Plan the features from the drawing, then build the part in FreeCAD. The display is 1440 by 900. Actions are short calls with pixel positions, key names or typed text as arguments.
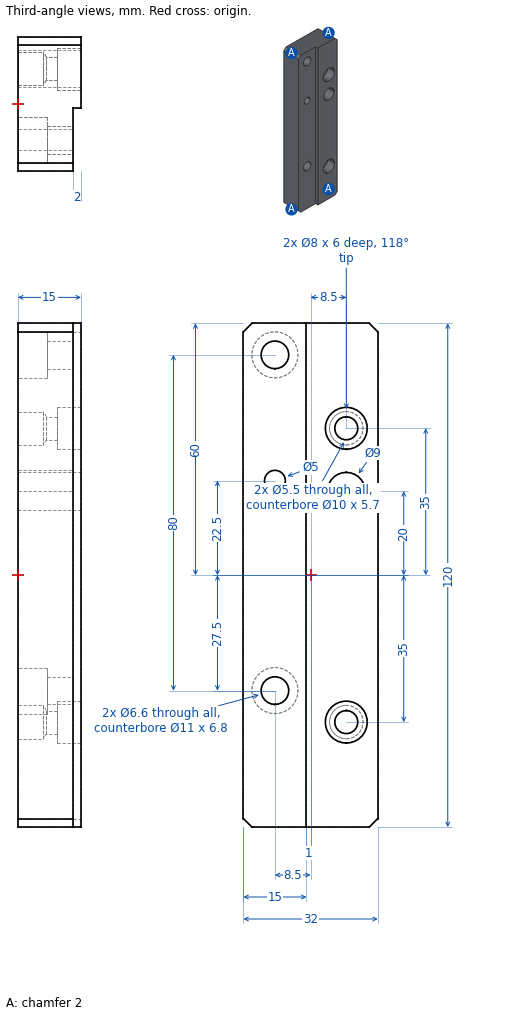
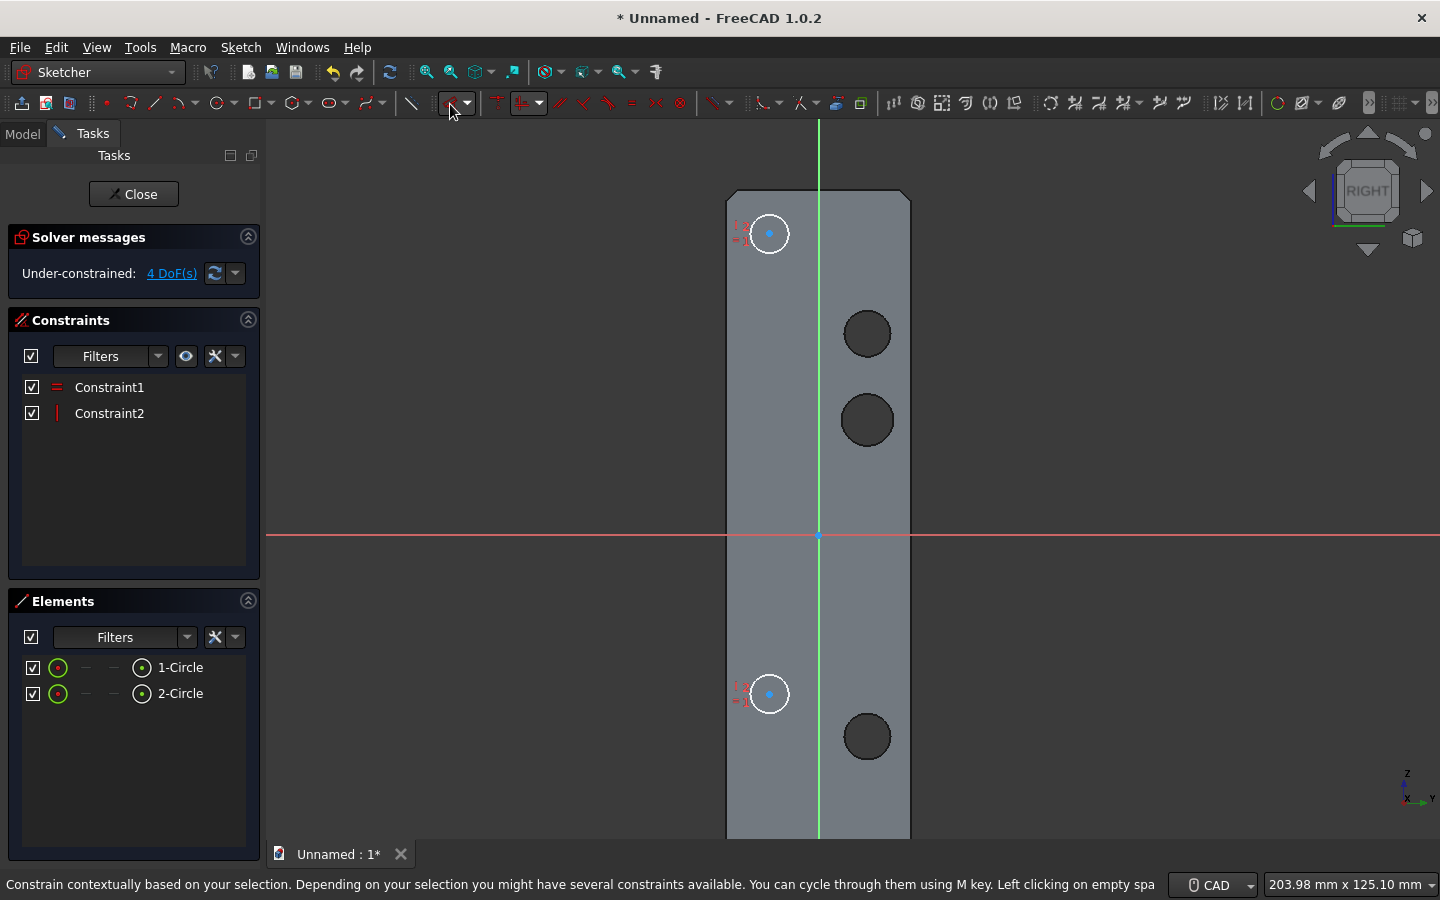
click(783, 681)
click(785, 646)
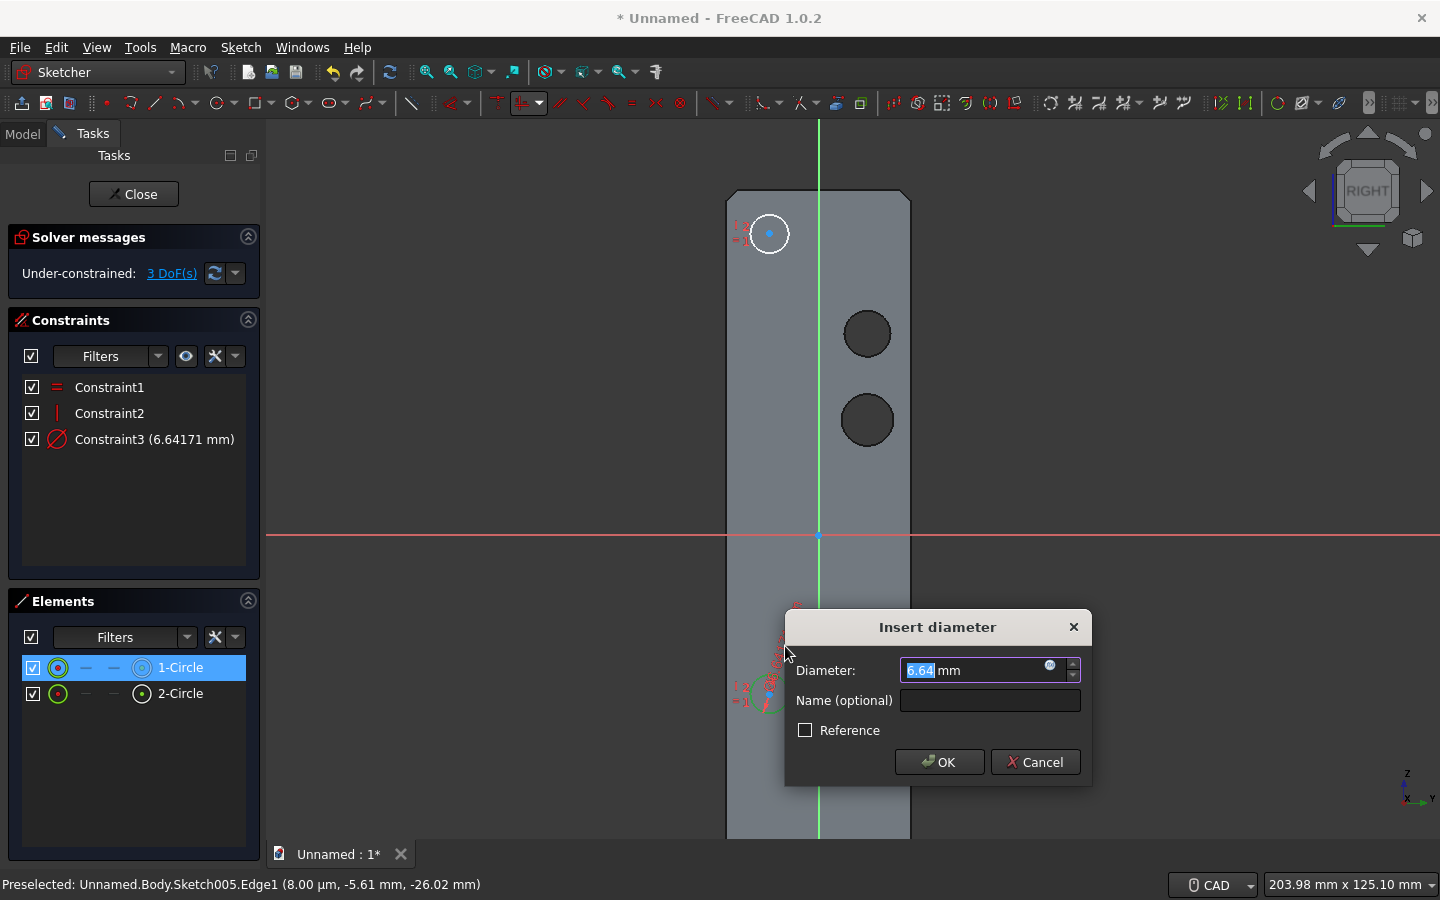
text(6.6)
key(Return)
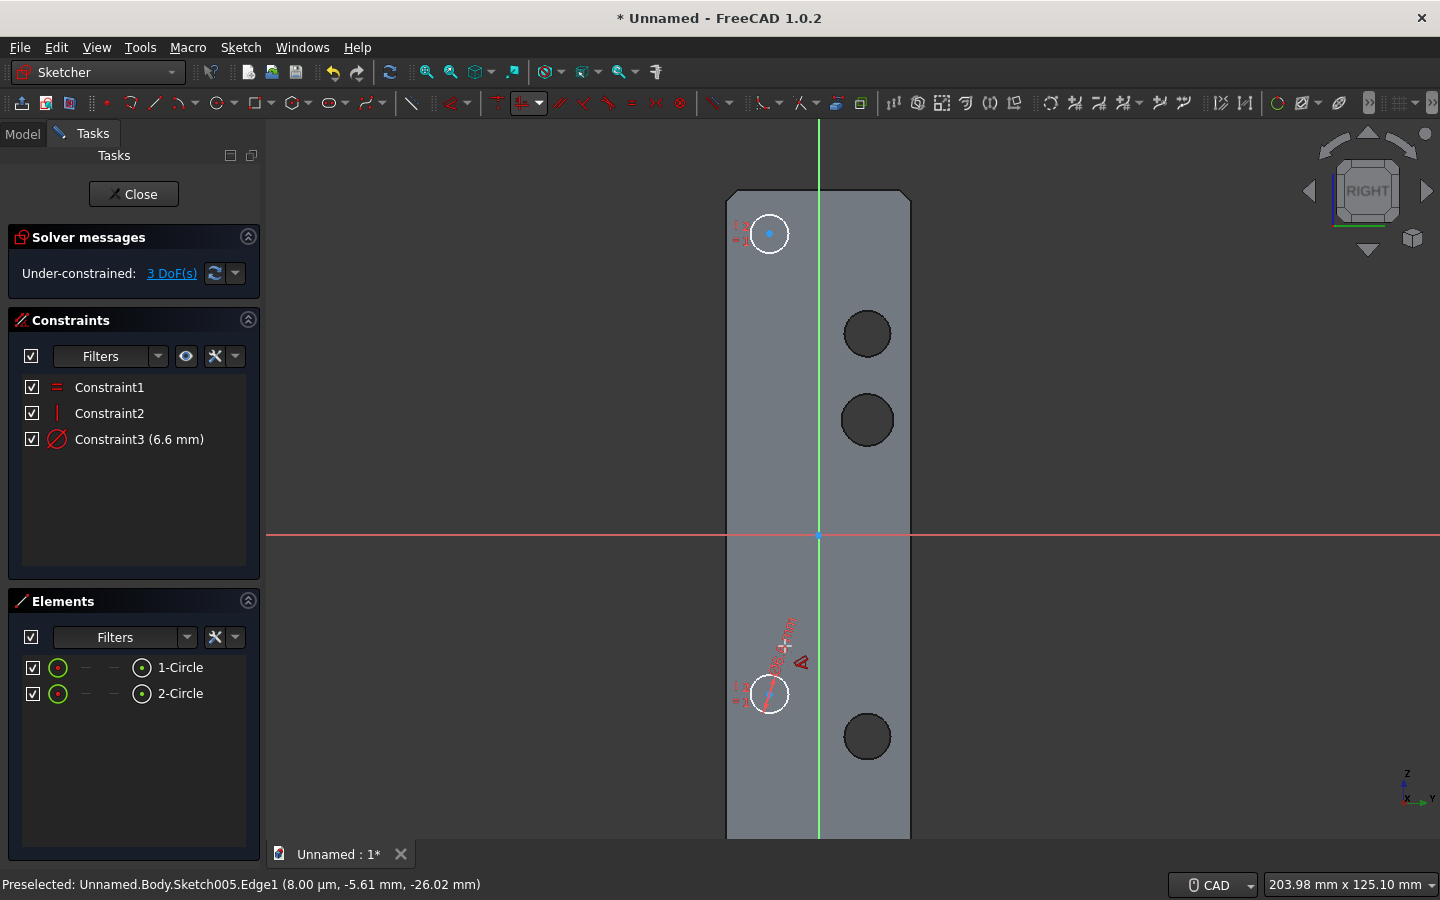
click(770, 694)
click(794, 728)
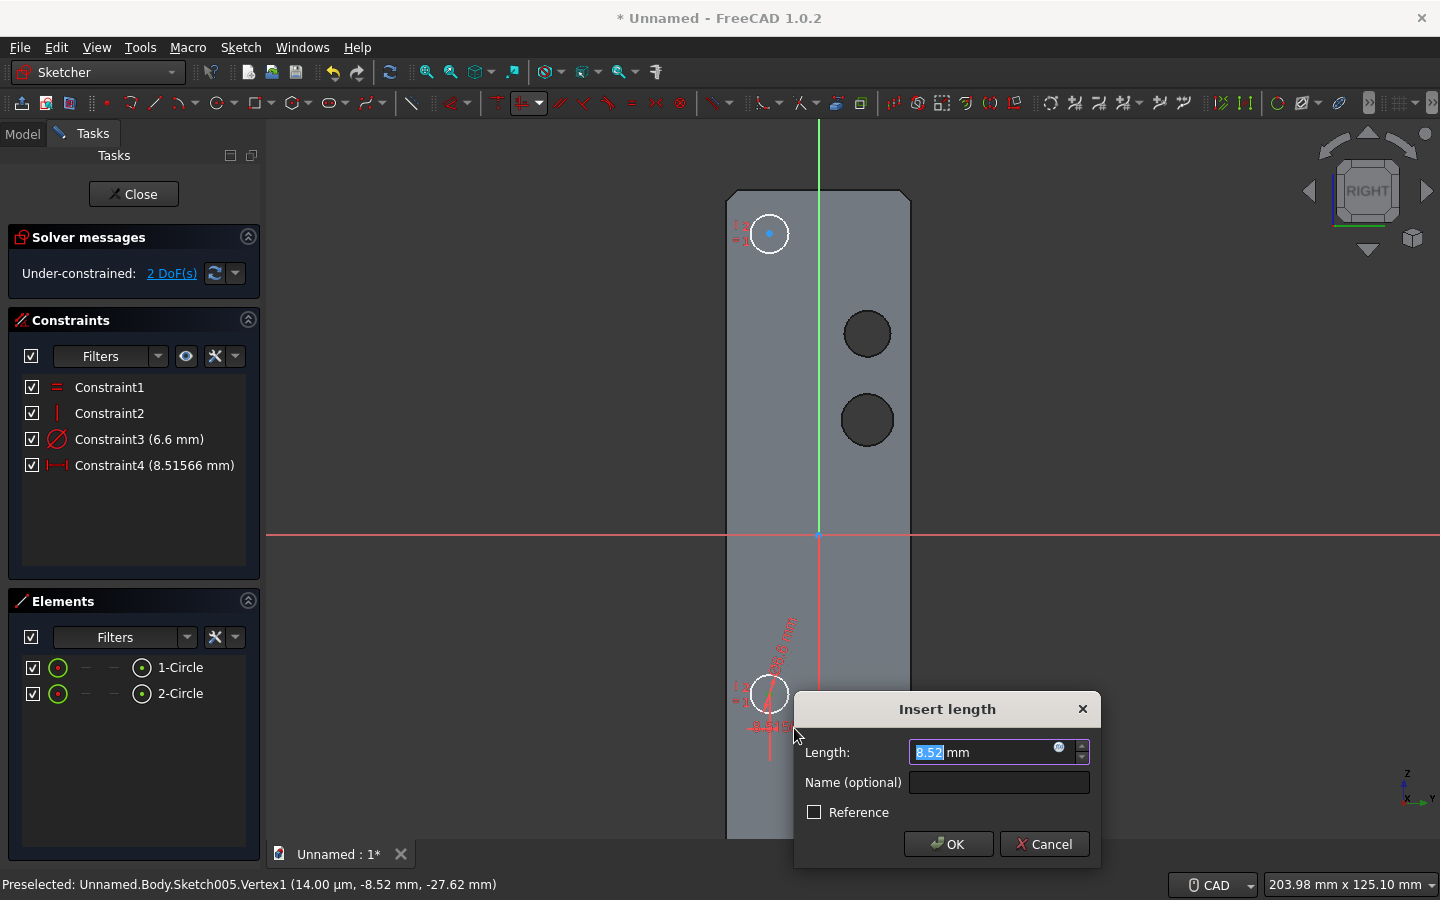
text(8.5)
key(Return)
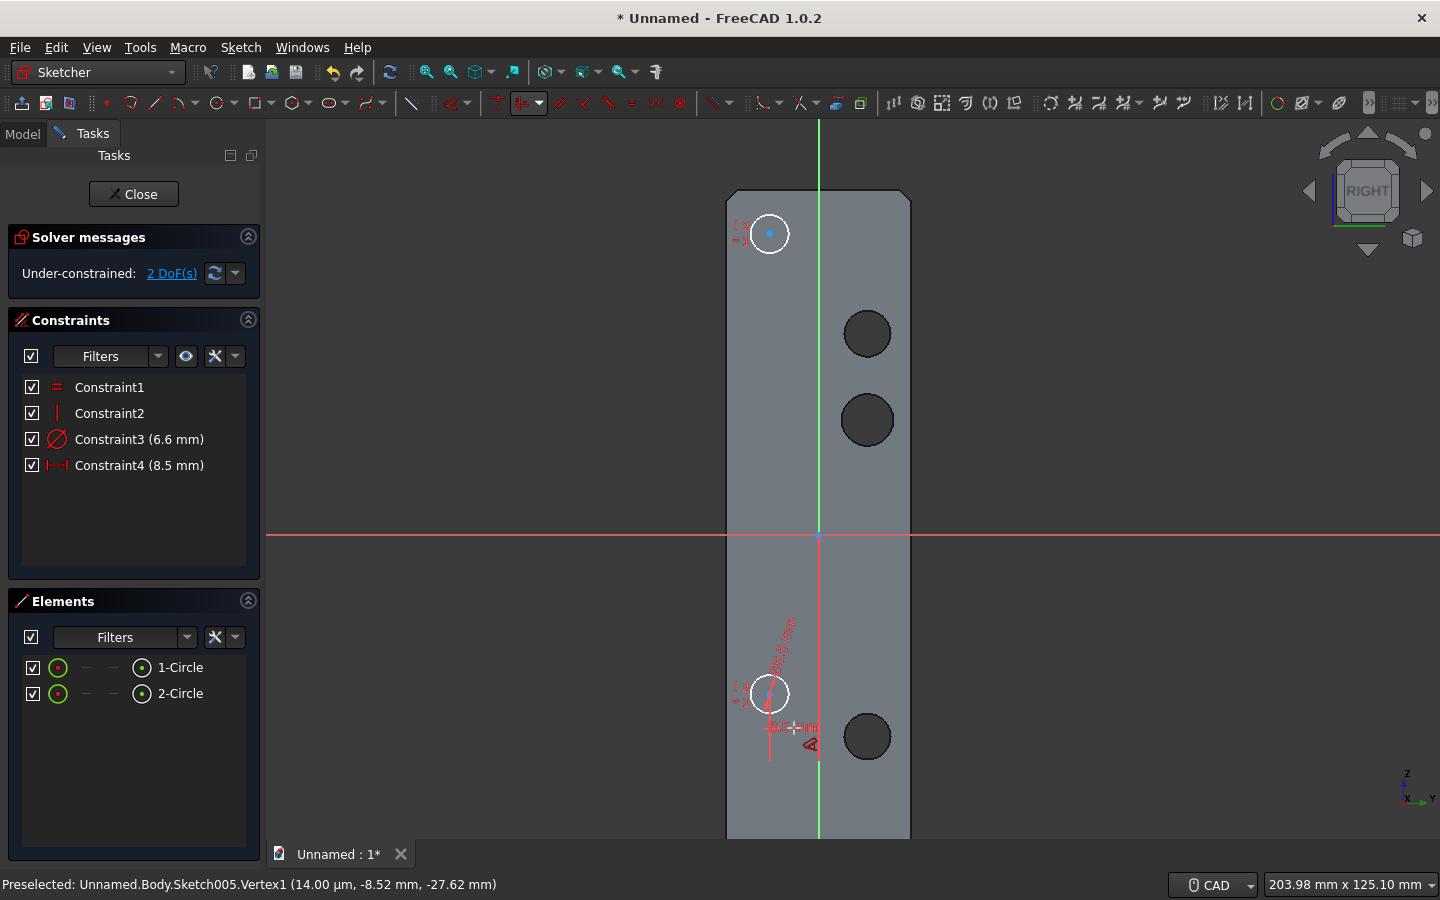
click(770, 694)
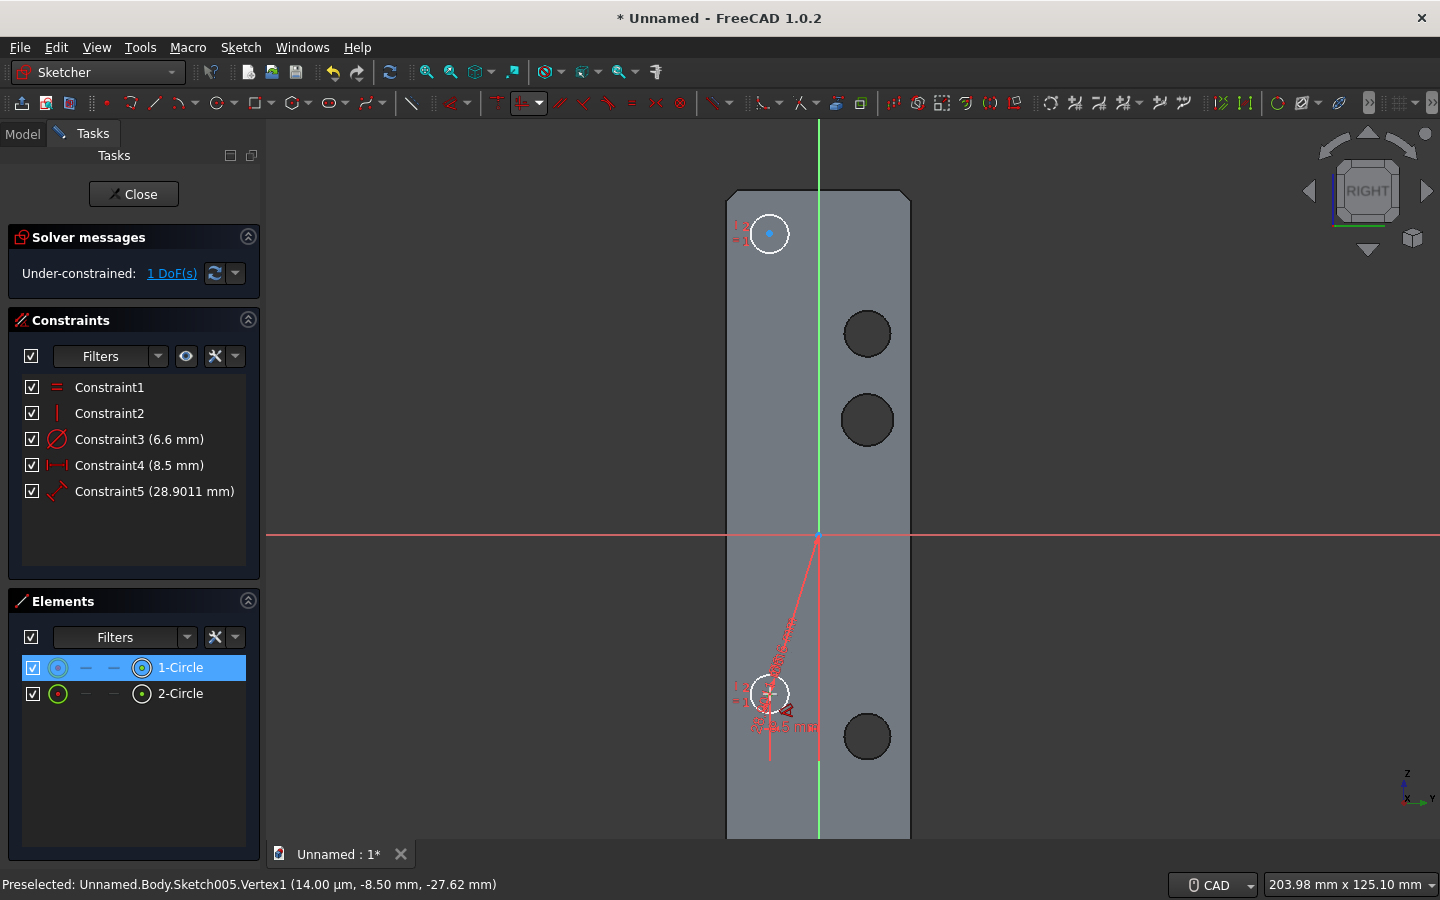
click(770, 234)
click(736, 464)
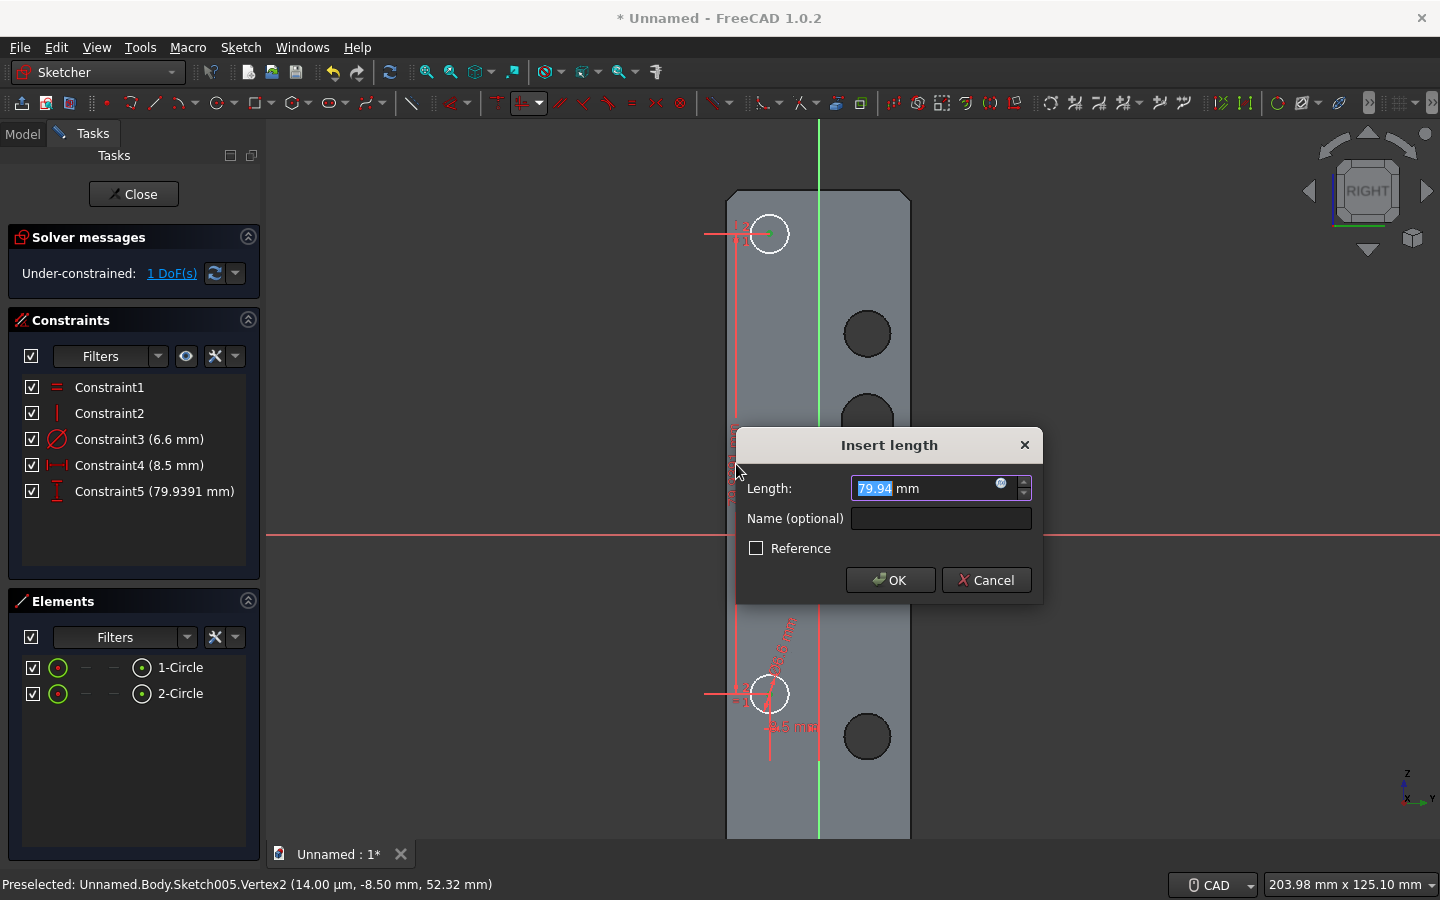
text(80)
key(Return)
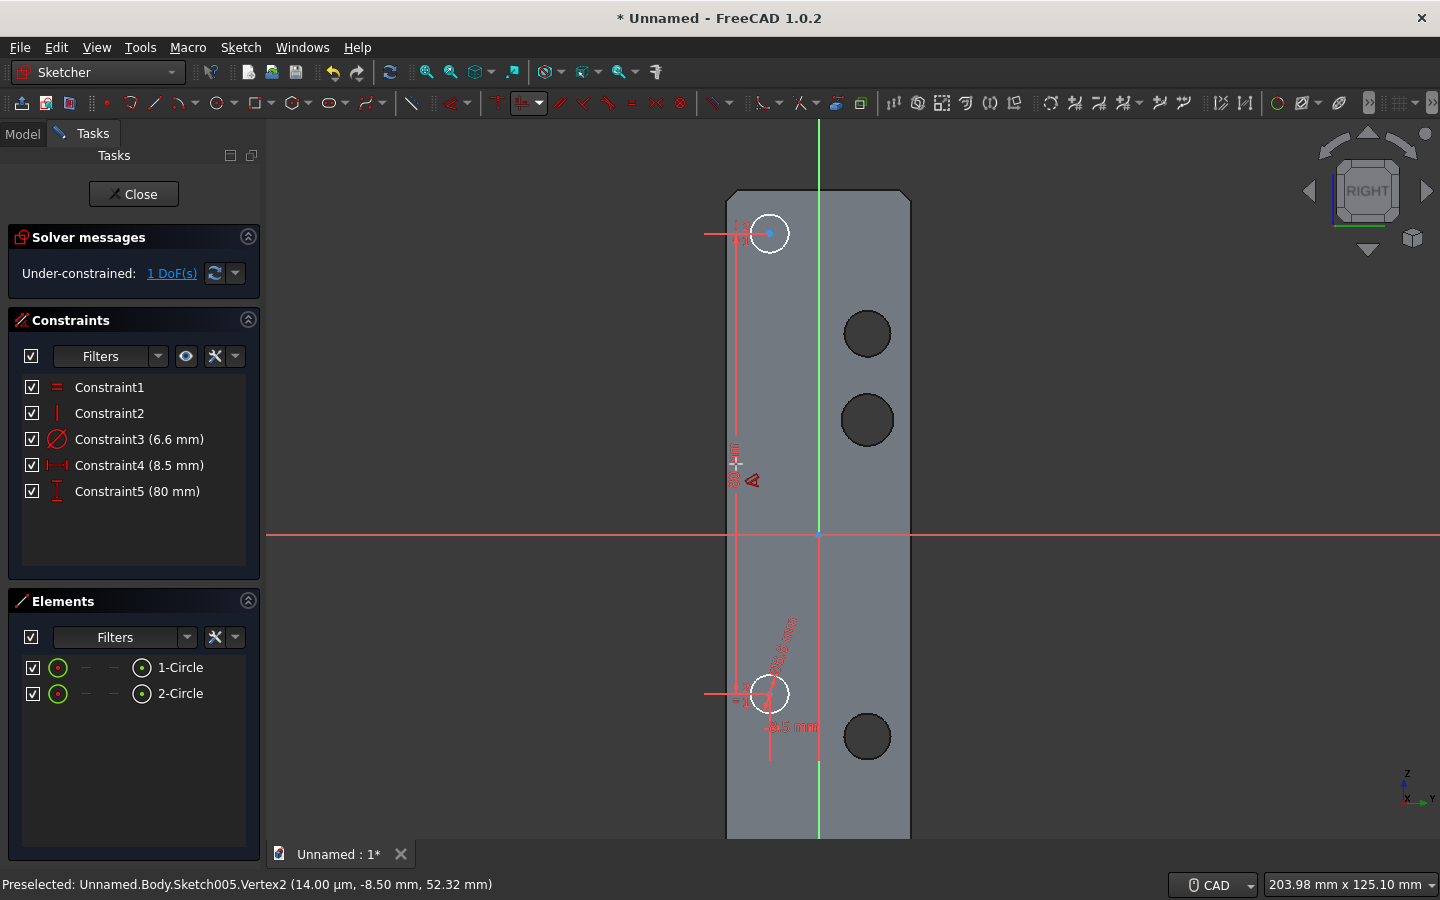
click(770, 694)
click(853, 615)